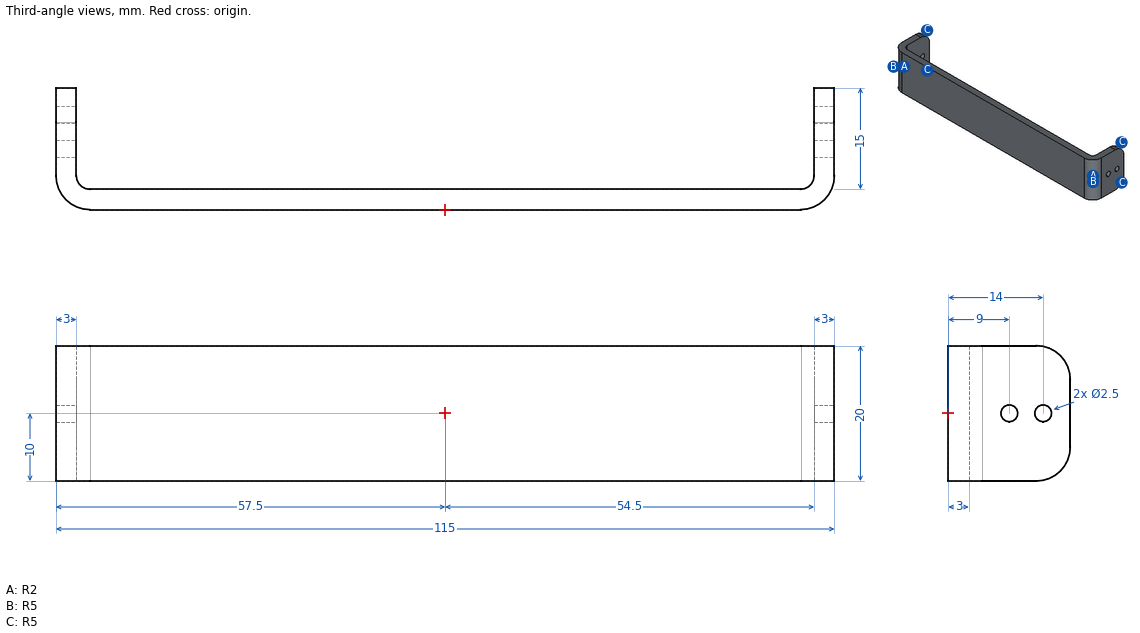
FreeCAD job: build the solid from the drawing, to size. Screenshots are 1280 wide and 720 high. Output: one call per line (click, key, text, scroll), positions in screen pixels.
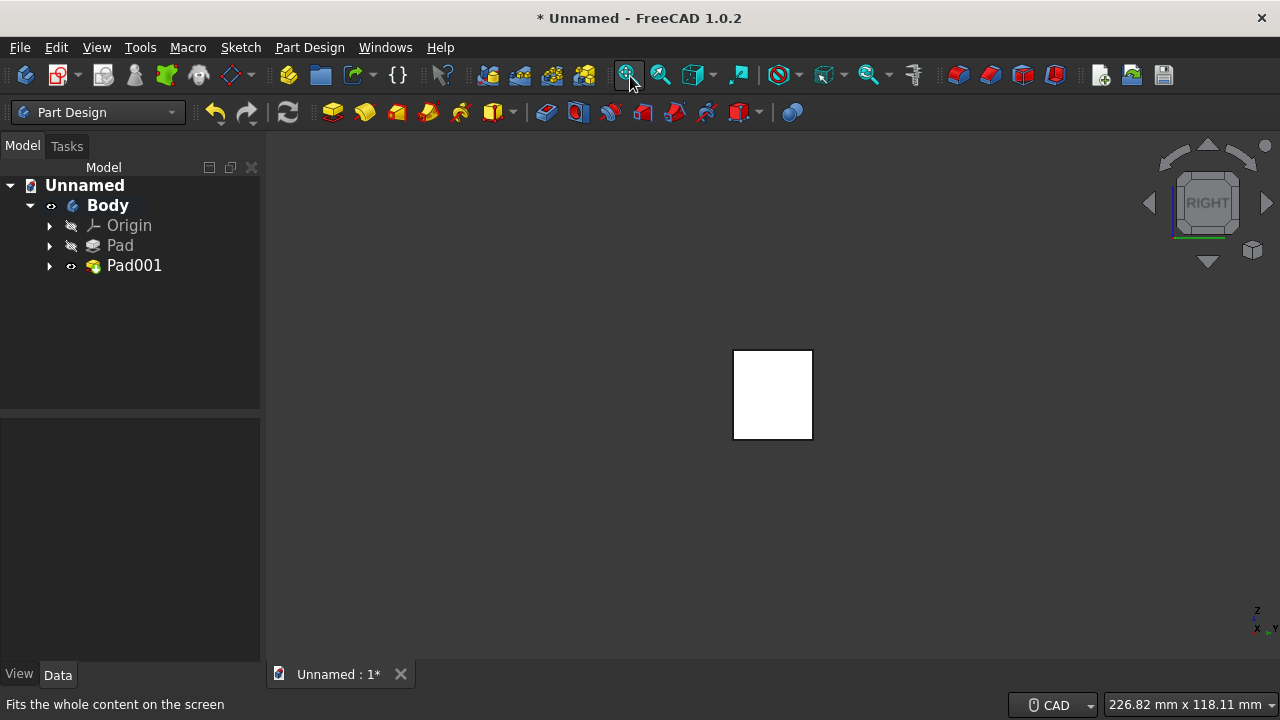
key(5)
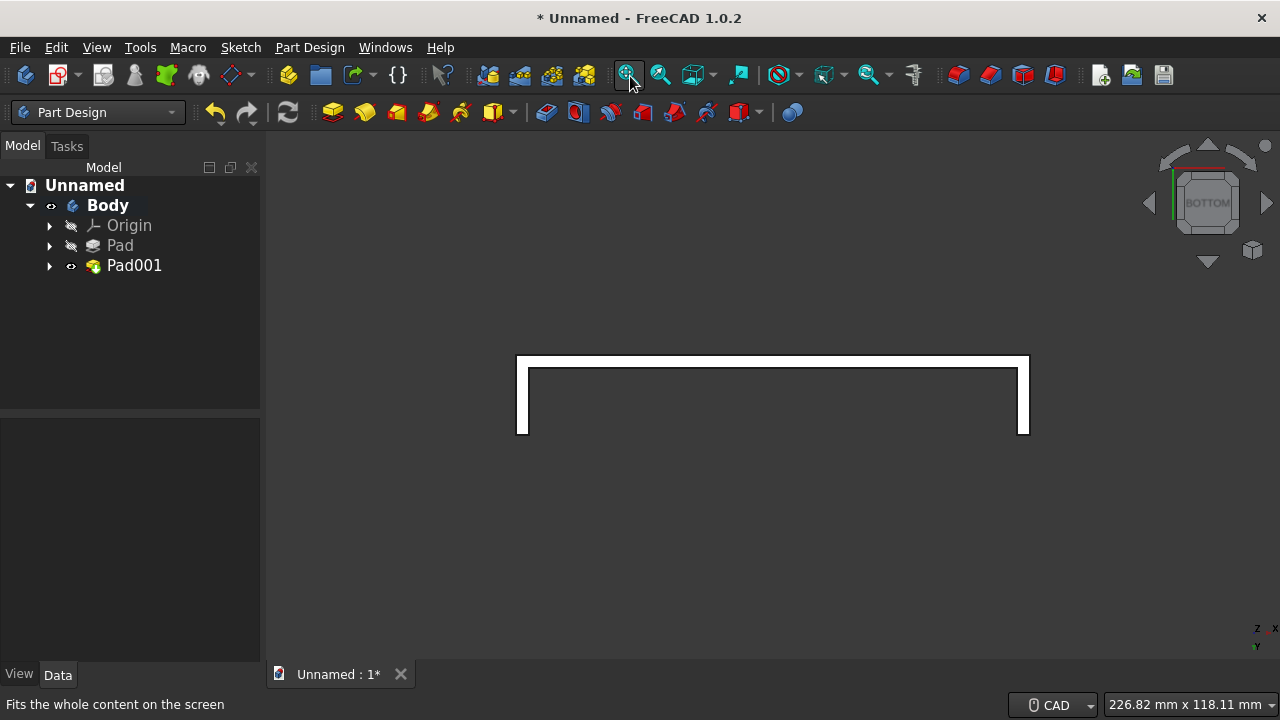
key(4)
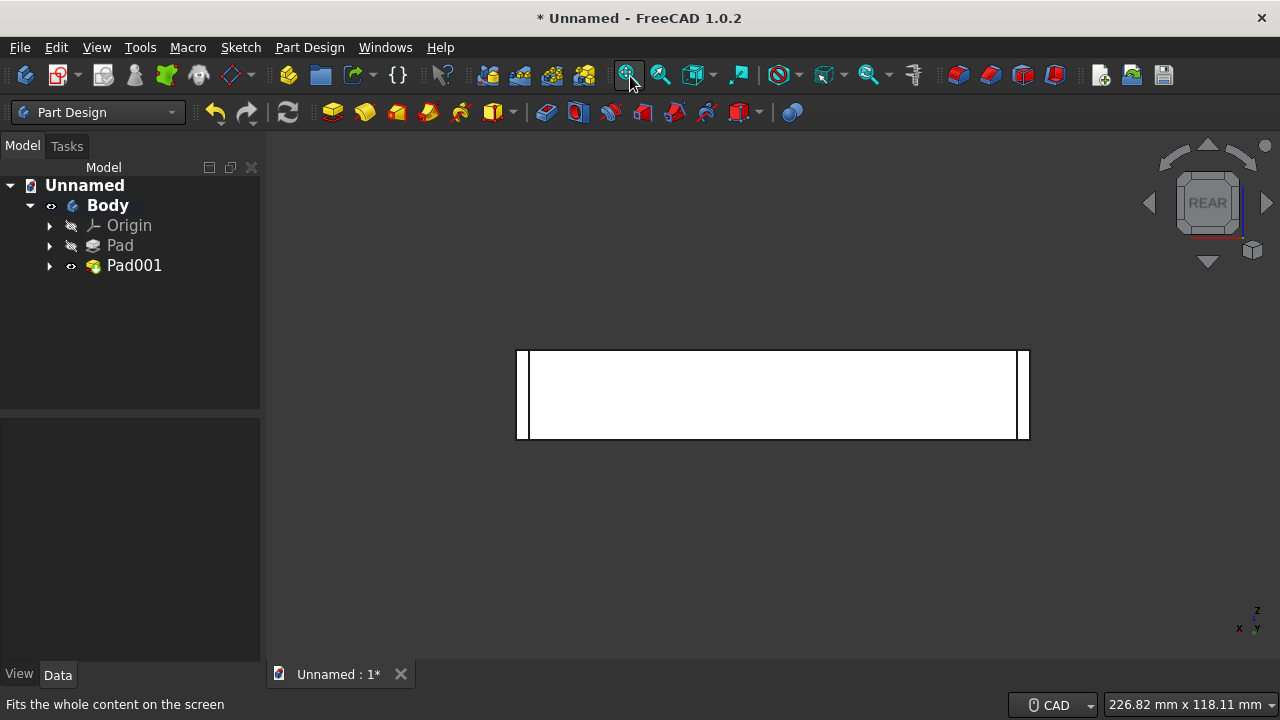
key(6)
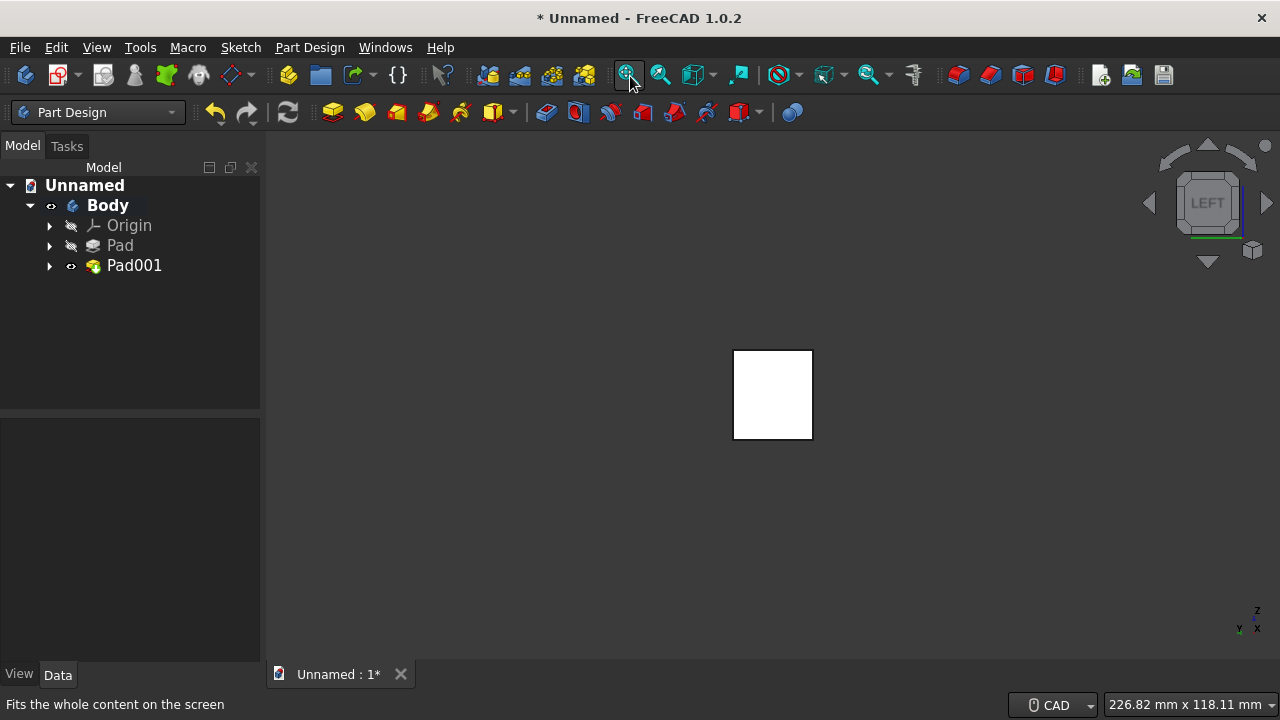
key(v)
key(f)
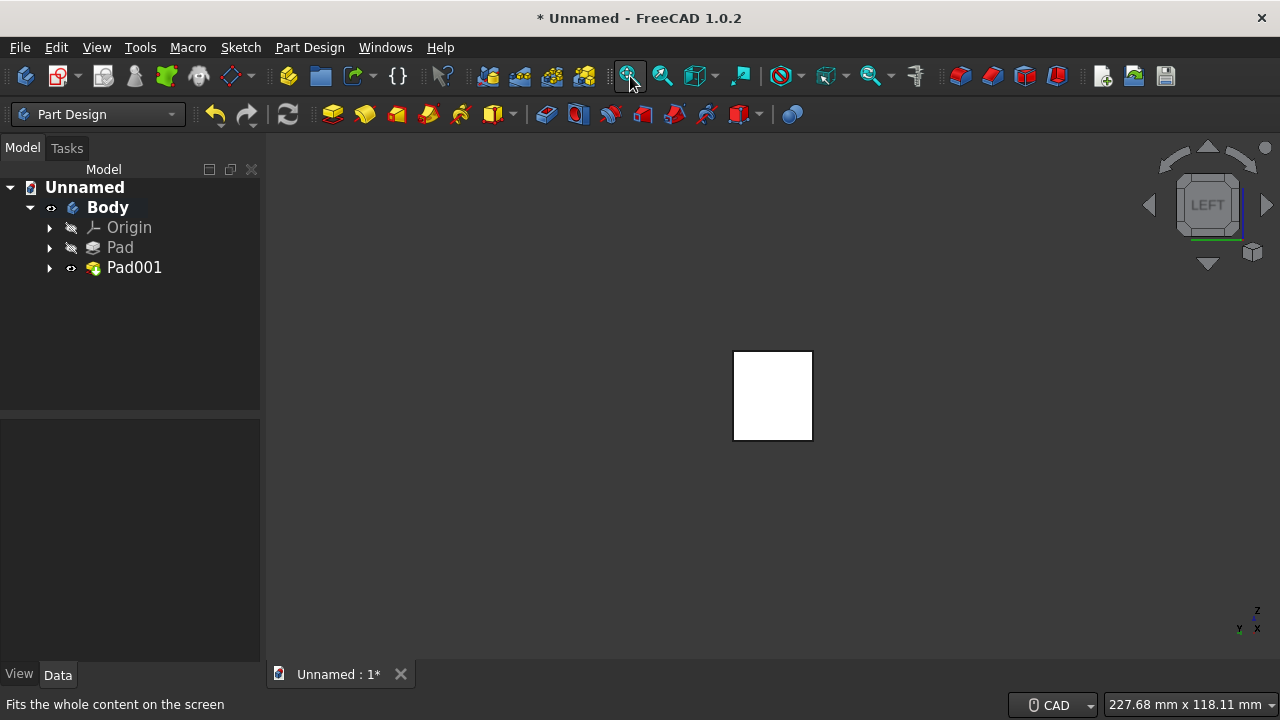
key(v)
key(3)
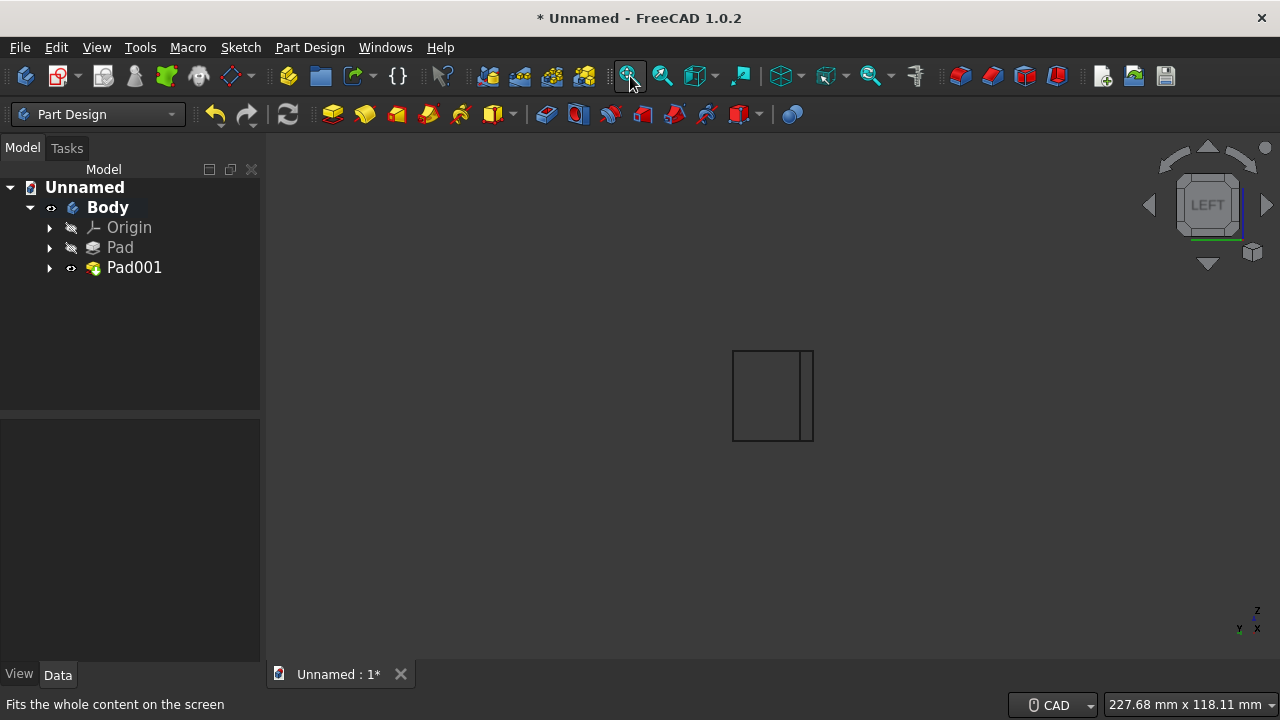
key(0)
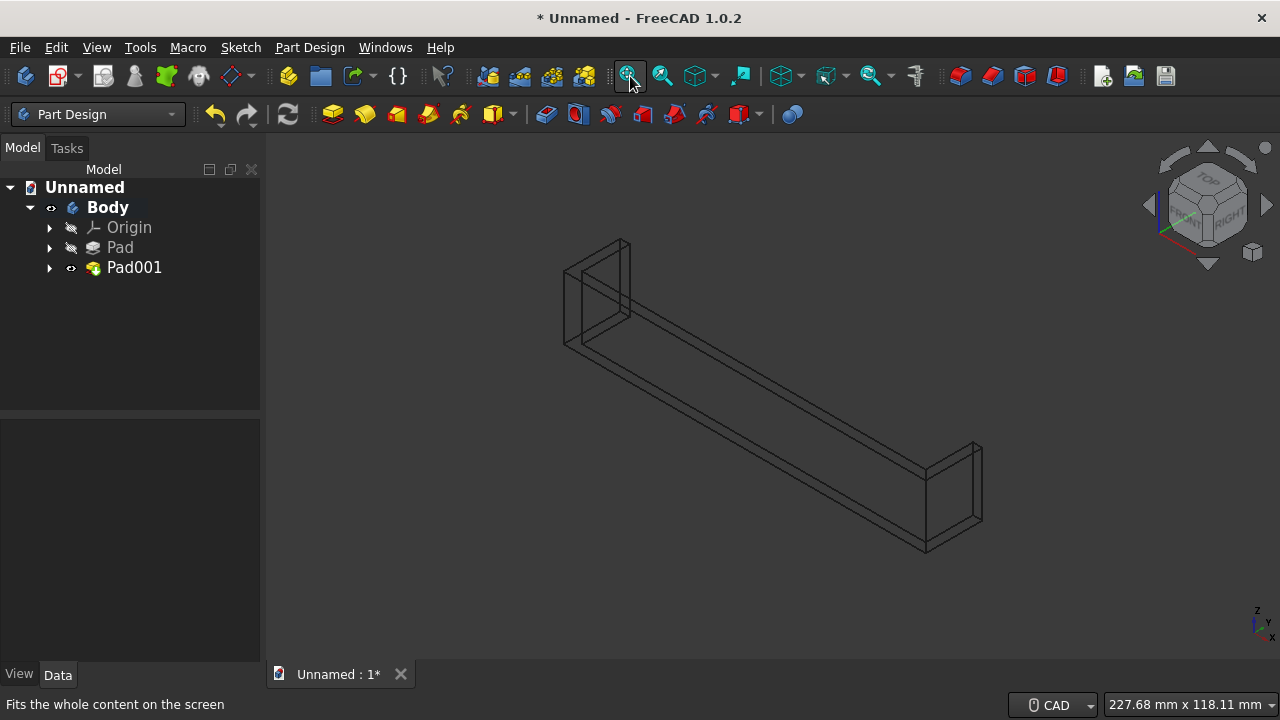
click(582, 307)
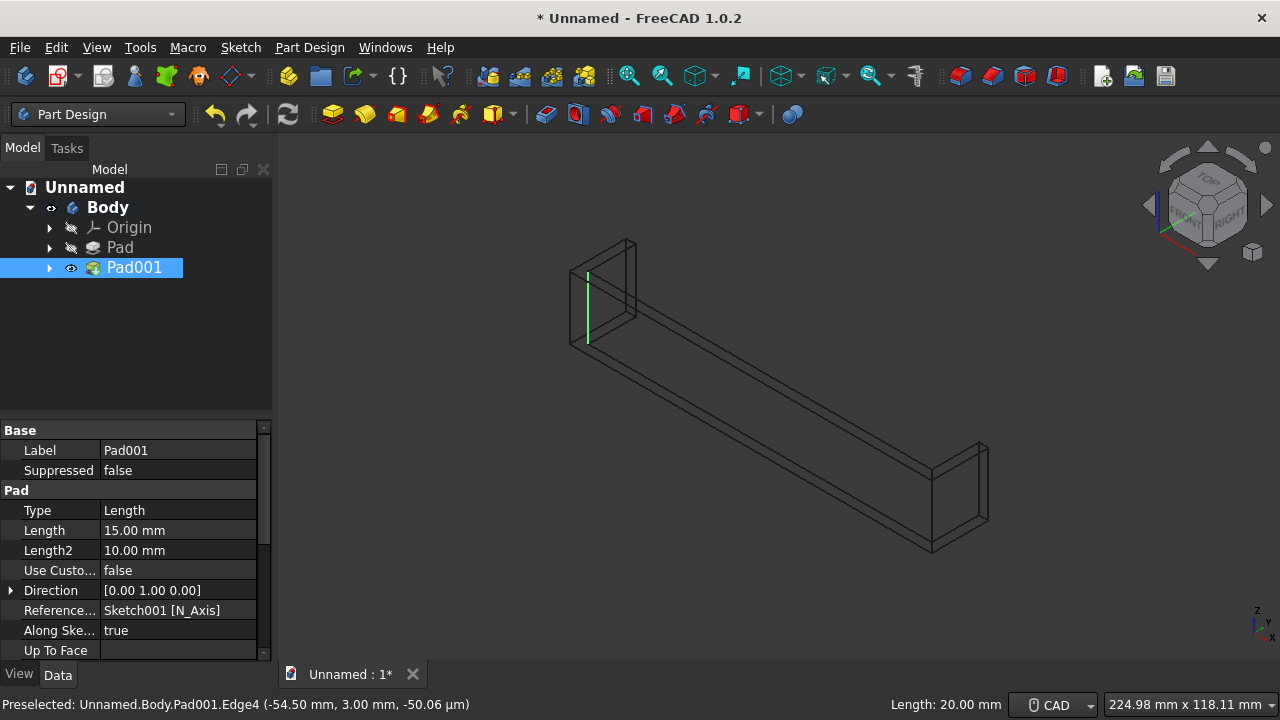
key(2)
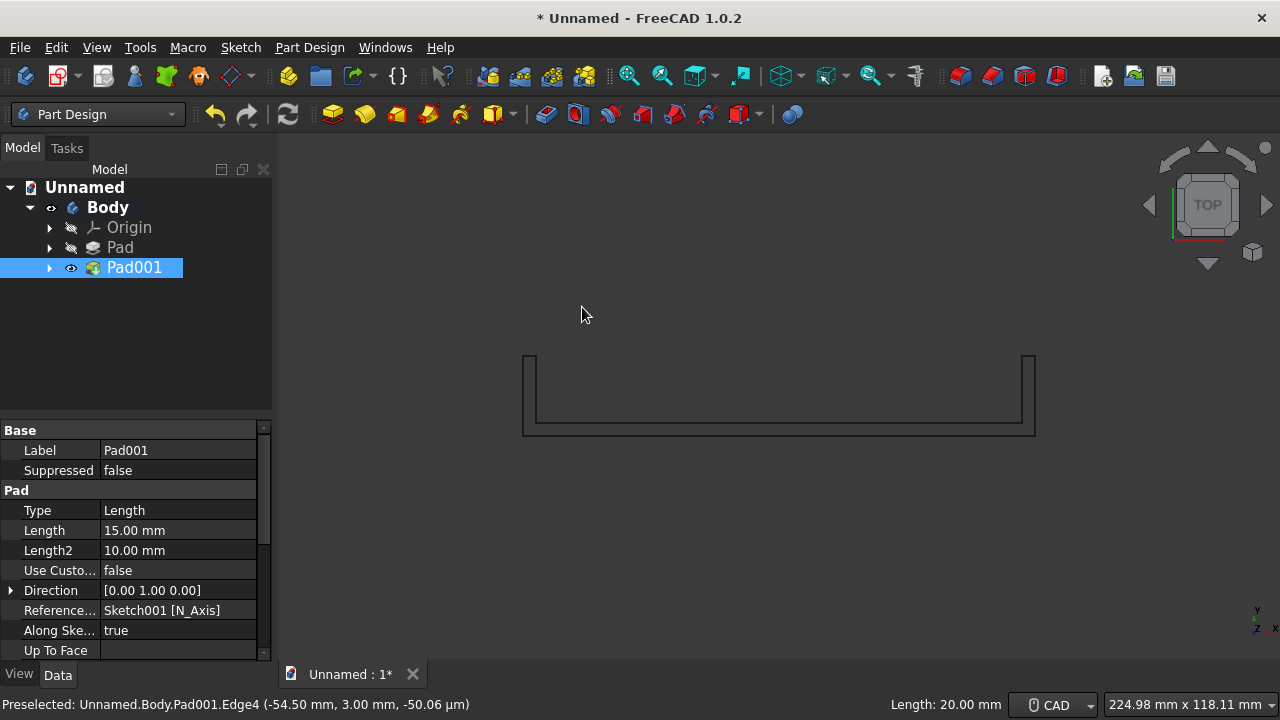
key(1)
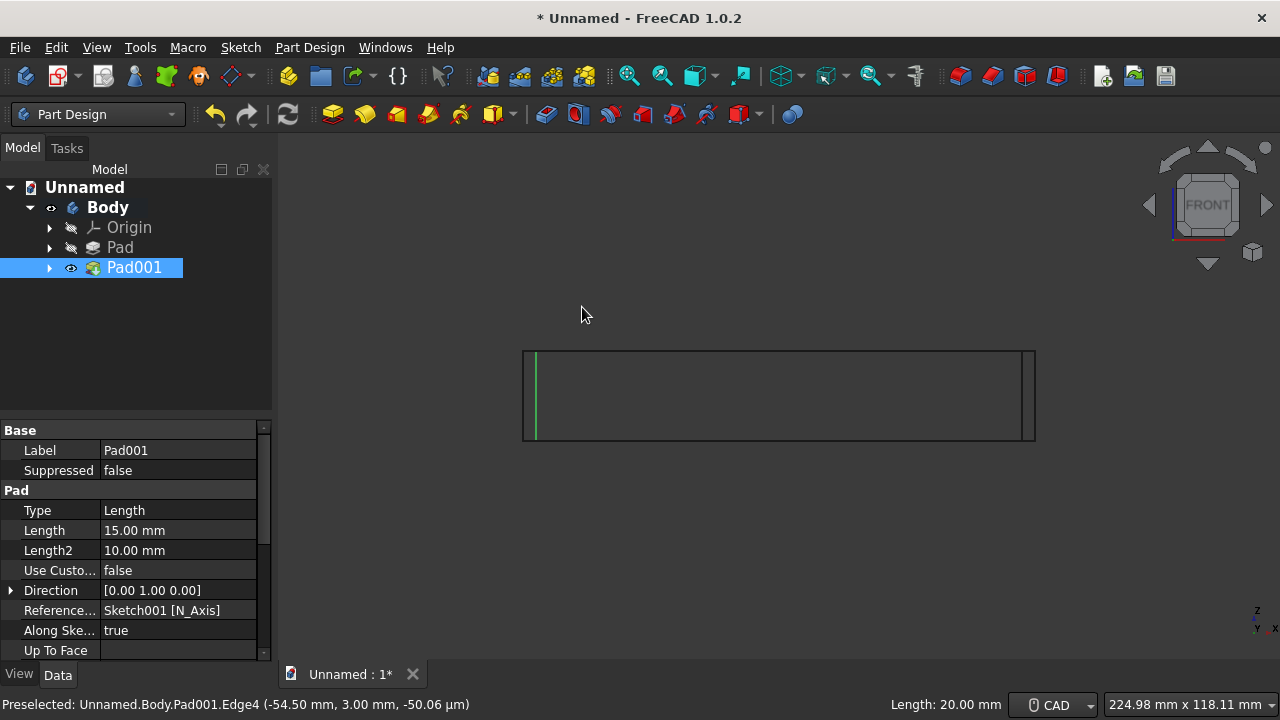
click(1022, 395, ctrl)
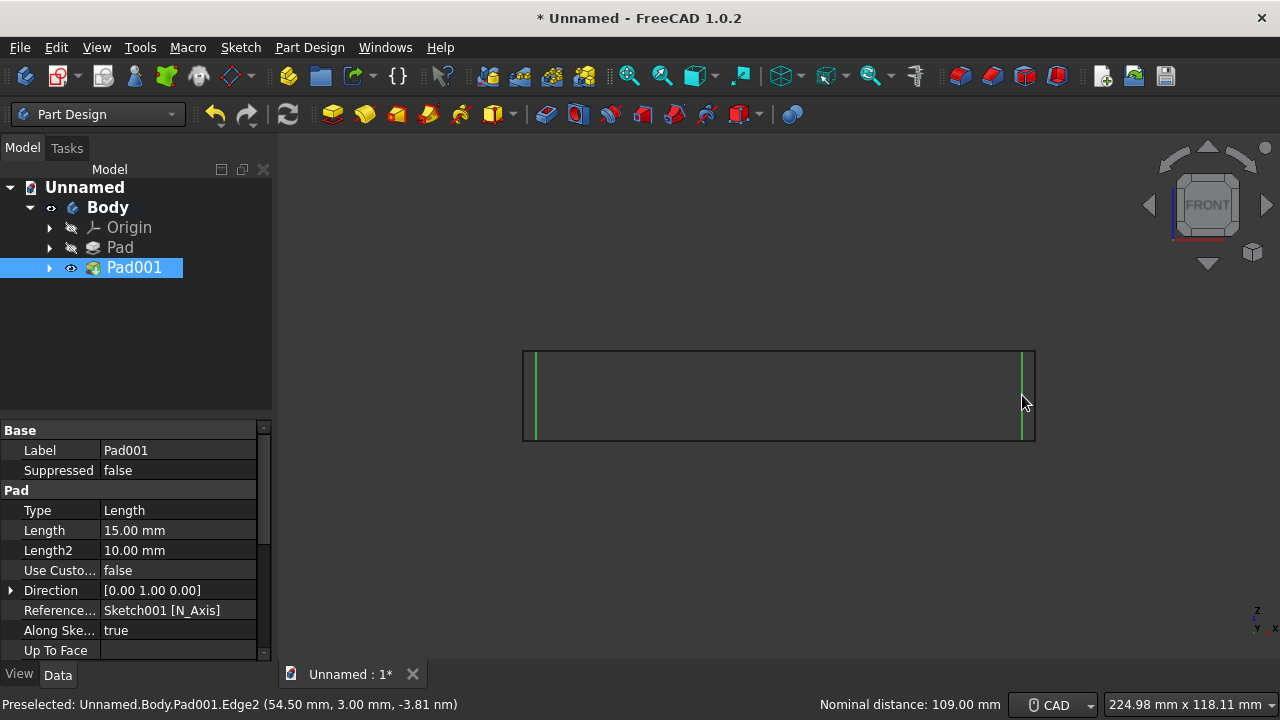
key(v)
key(1)